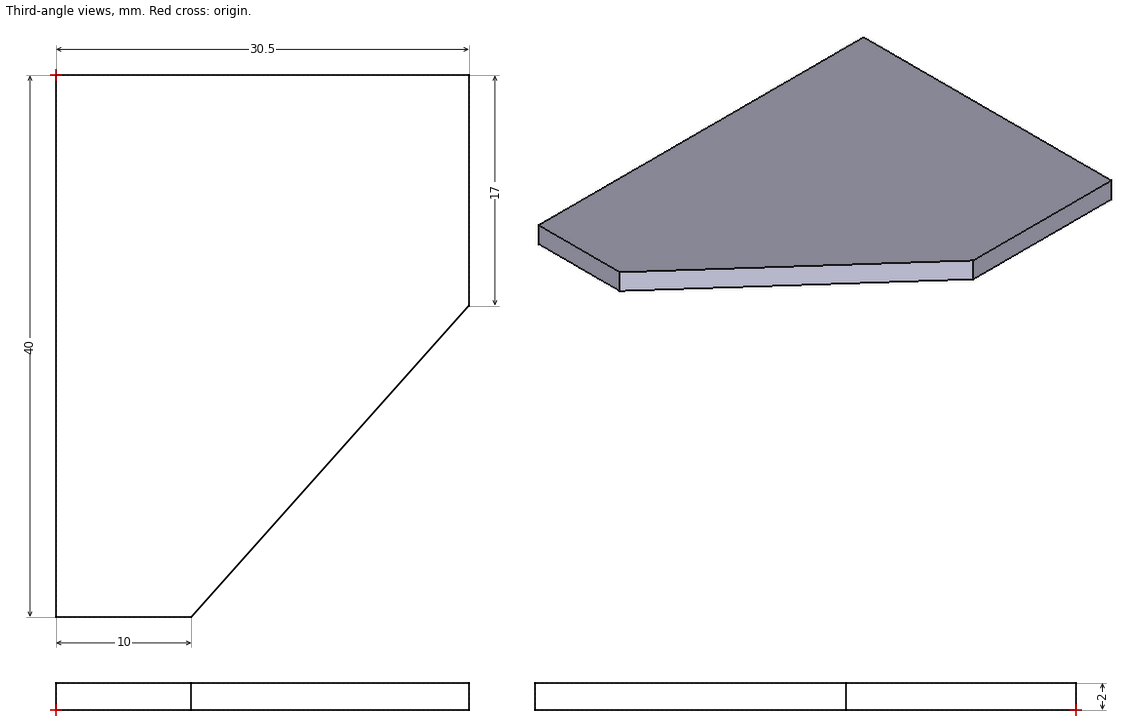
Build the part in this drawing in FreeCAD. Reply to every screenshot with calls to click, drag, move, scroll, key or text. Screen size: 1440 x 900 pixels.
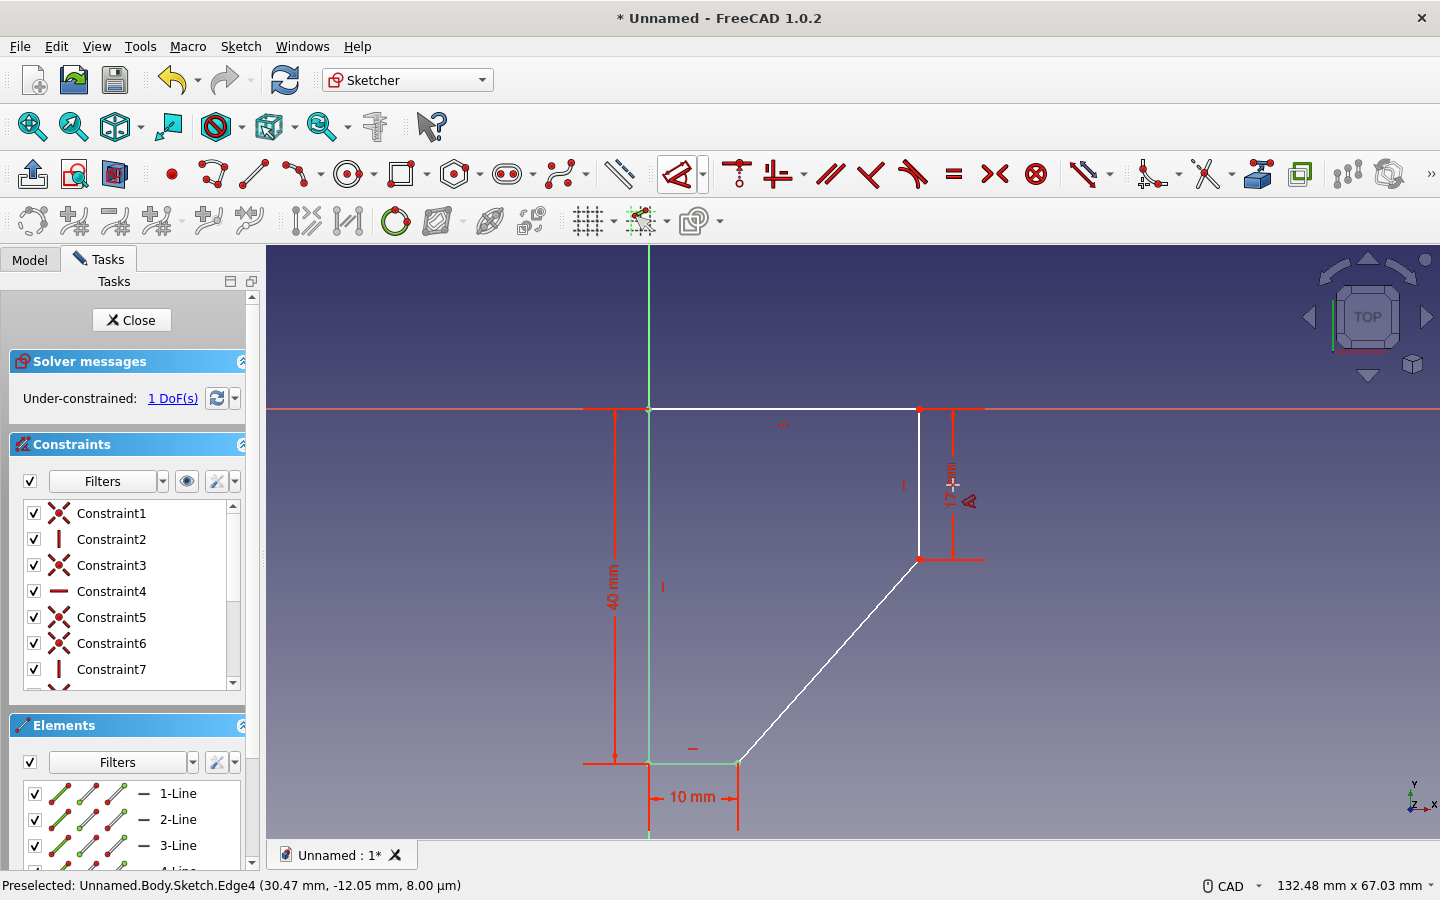
click(838, 409)
click(784, 375)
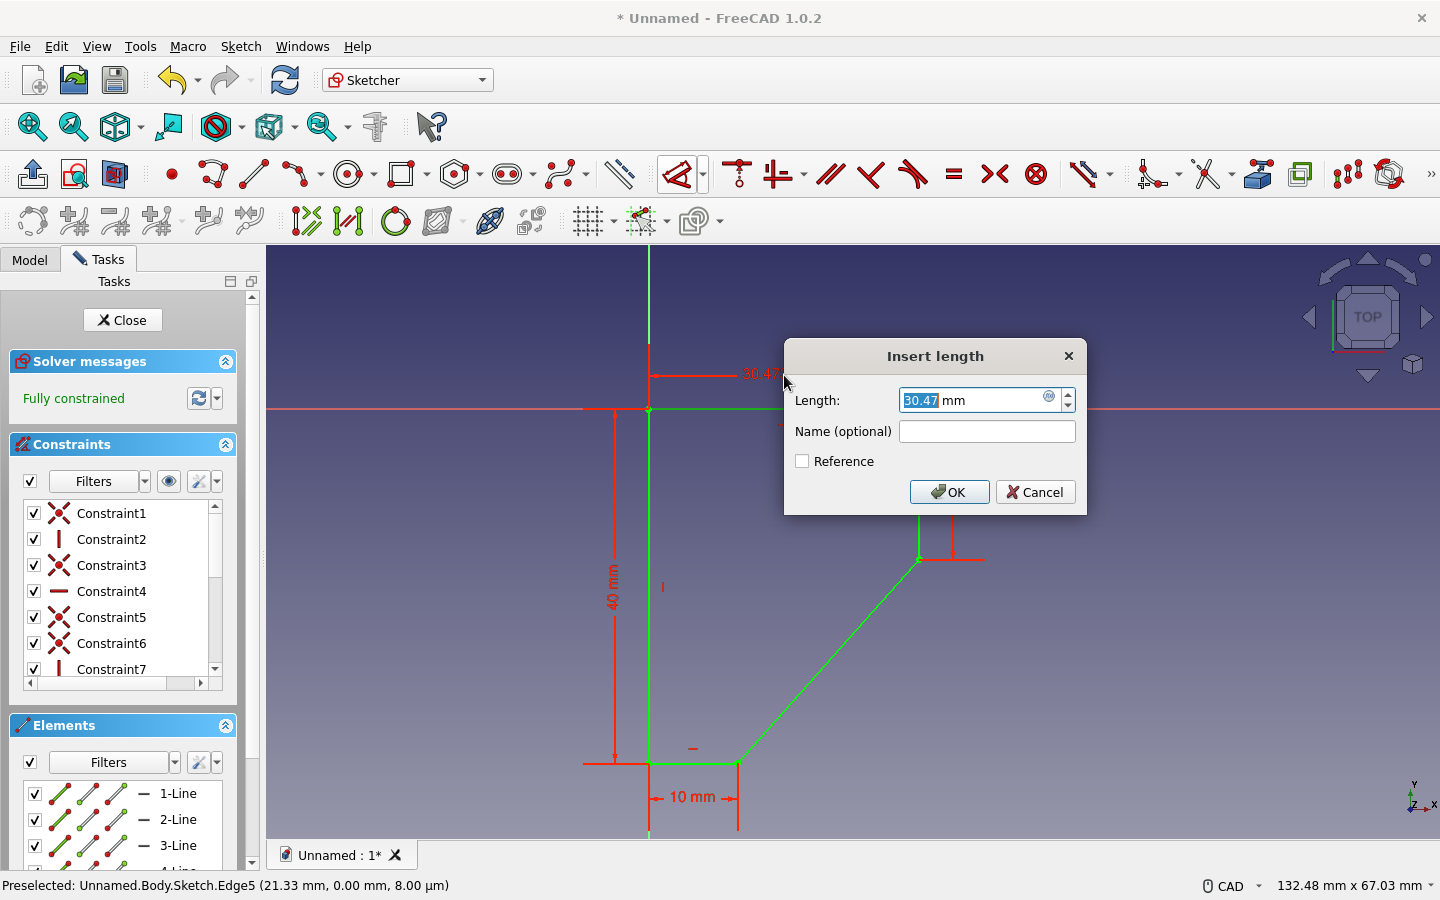
text(30.5)
key(Return)
key(Escape)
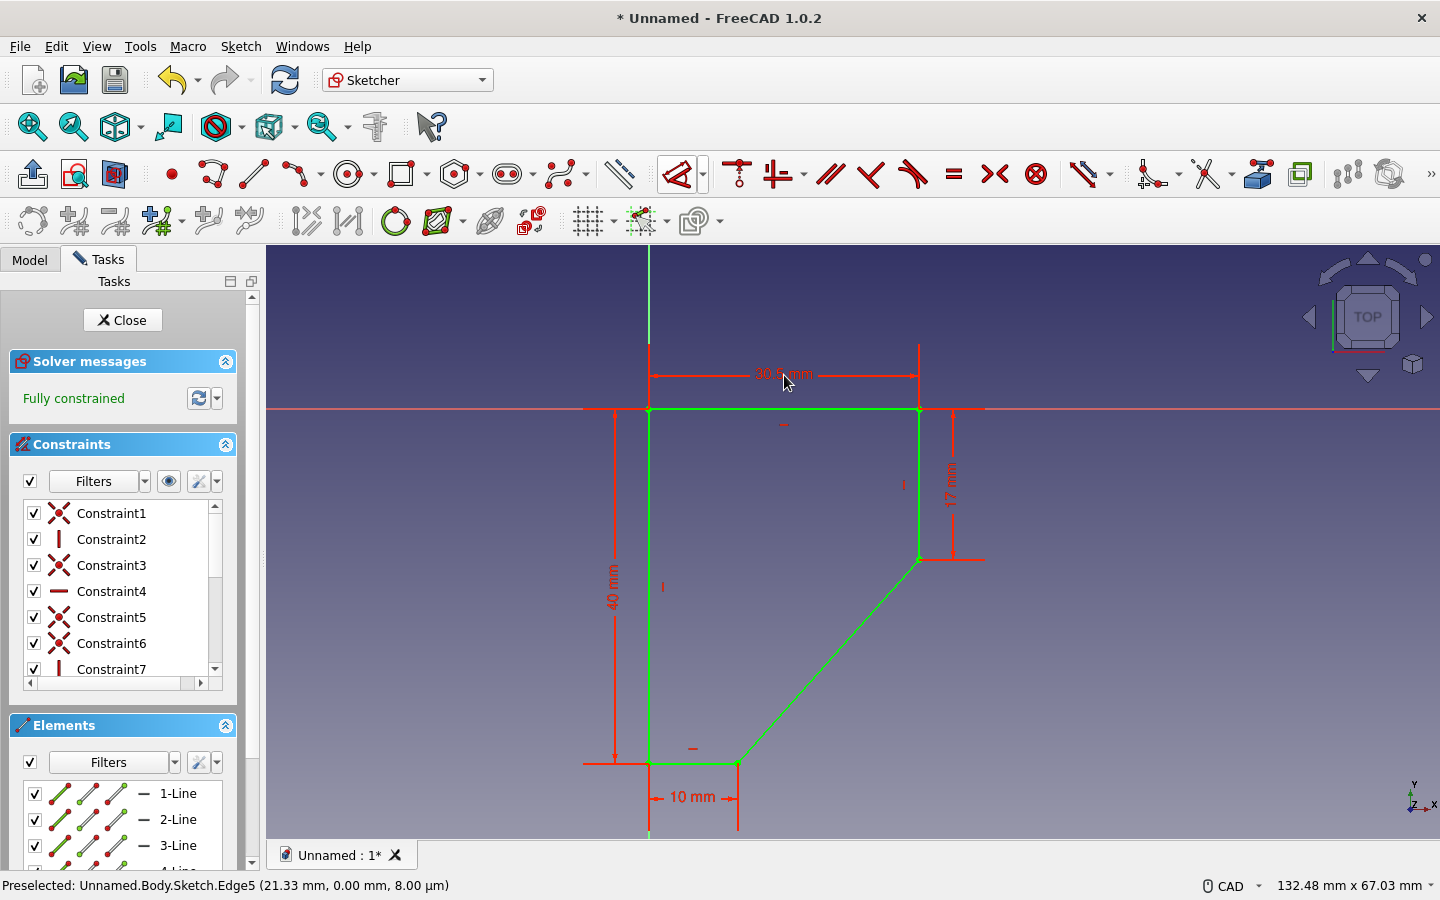
click(123, 320)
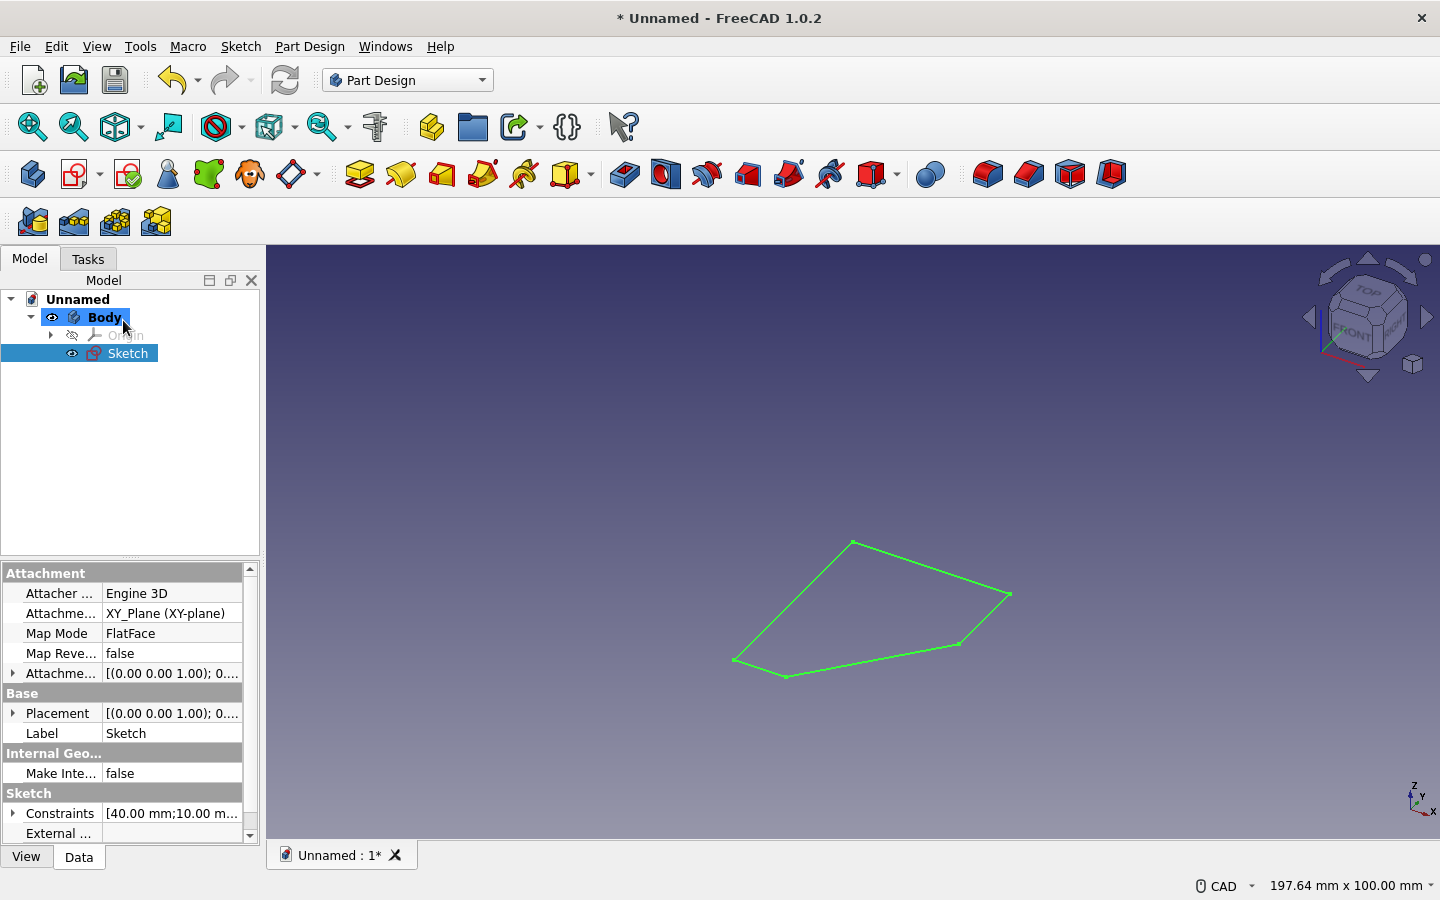
click(360, 174)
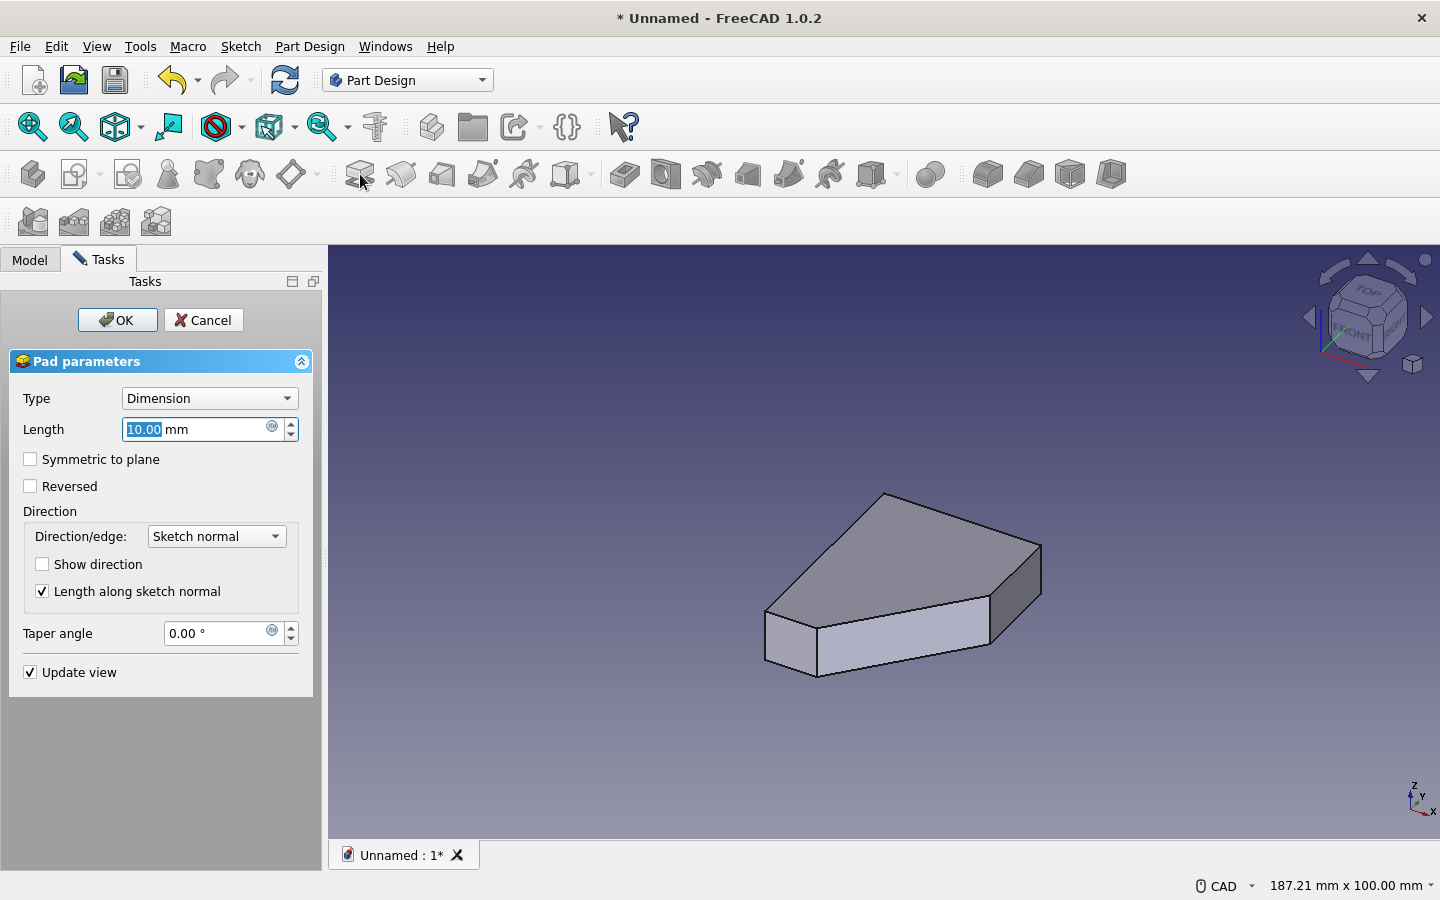
text(2)
key(Tab)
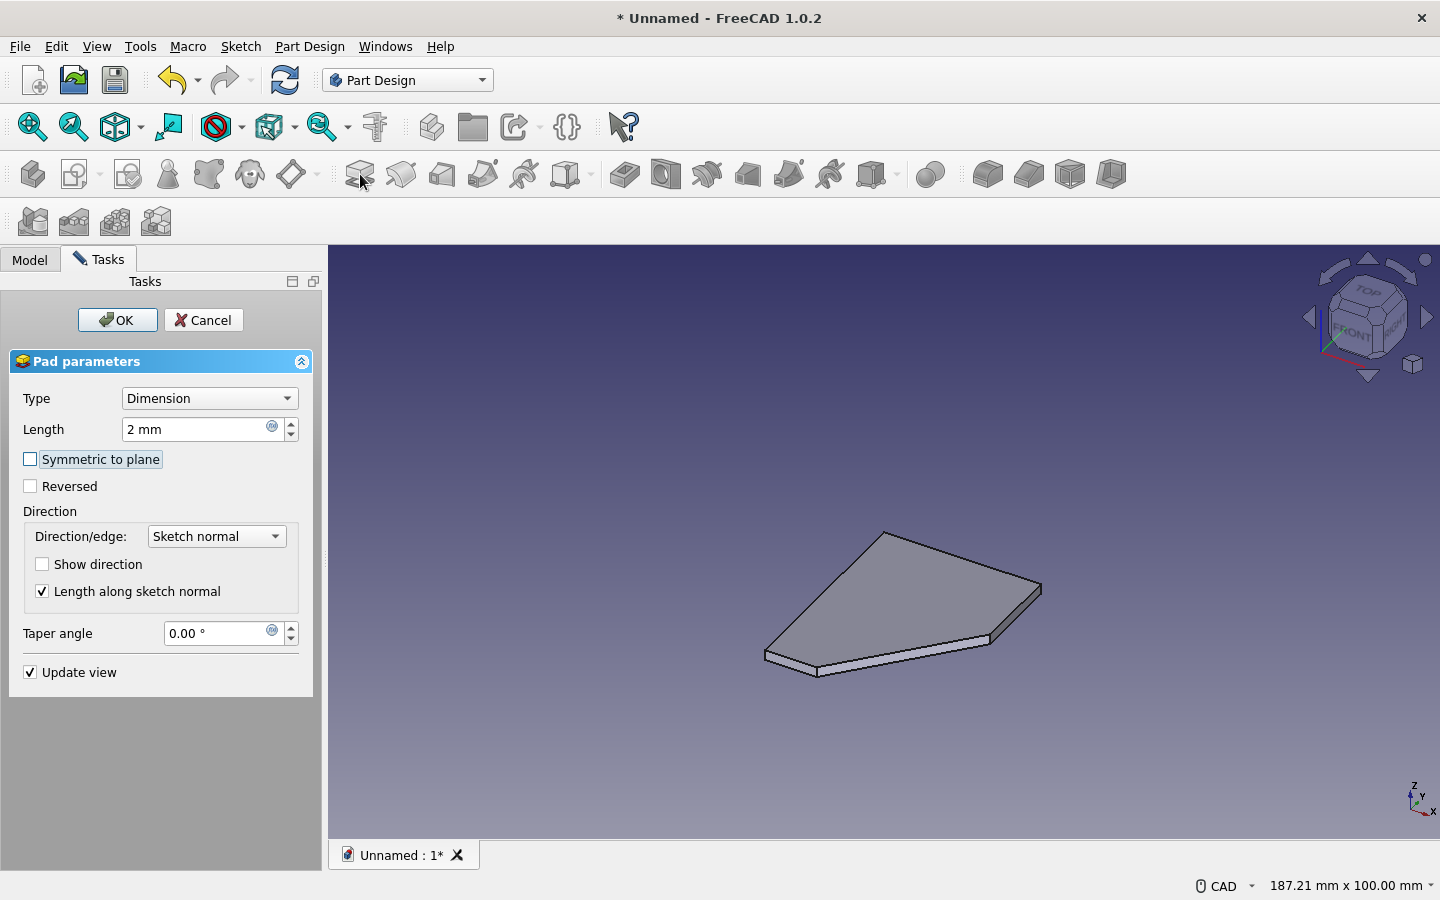
click(118, 320)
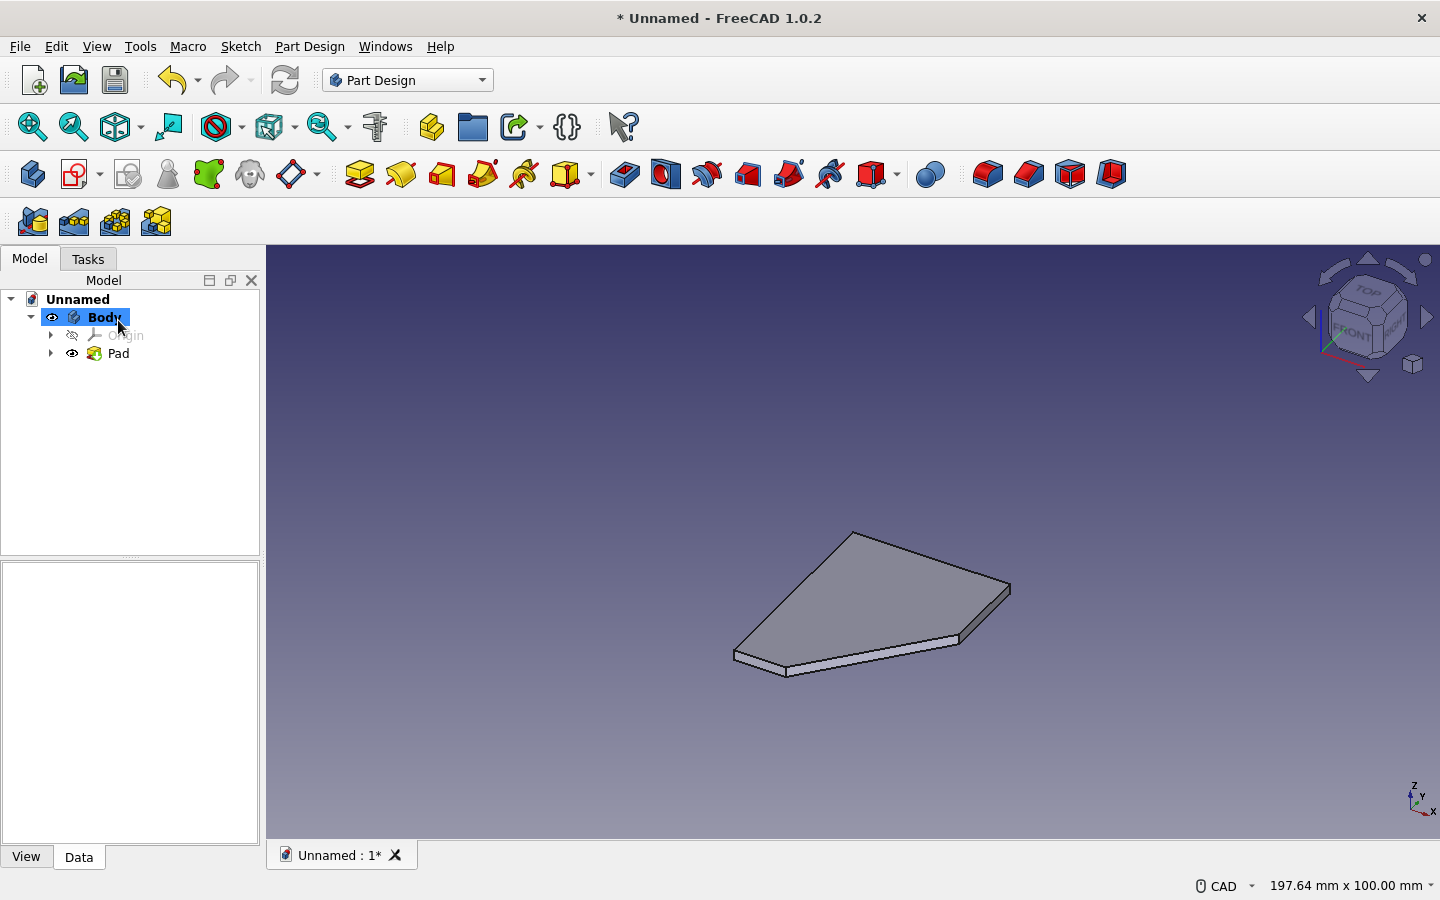
key(0)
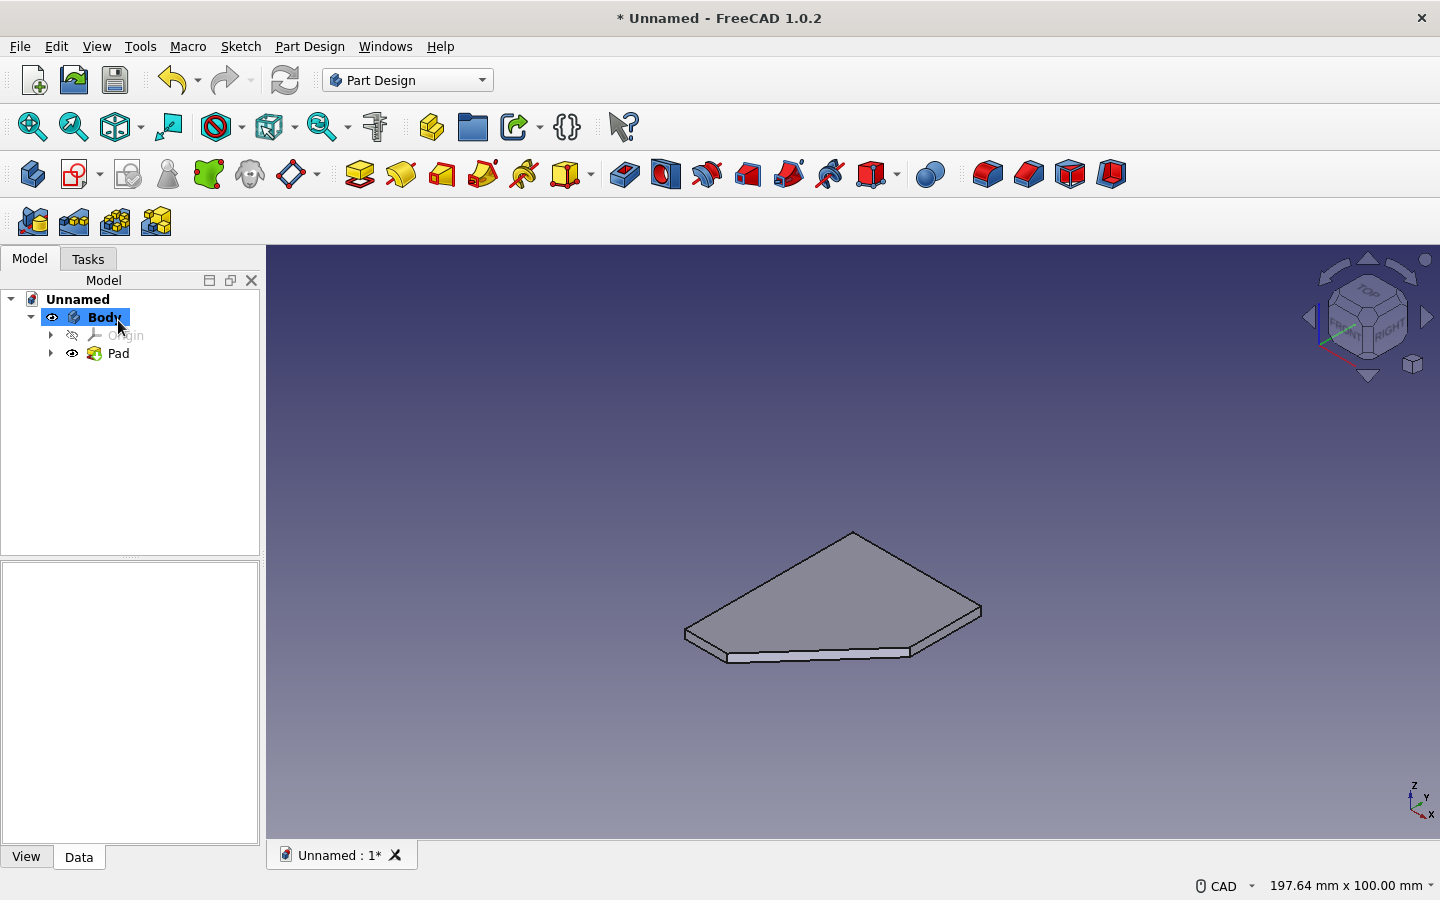
click(33, 128)